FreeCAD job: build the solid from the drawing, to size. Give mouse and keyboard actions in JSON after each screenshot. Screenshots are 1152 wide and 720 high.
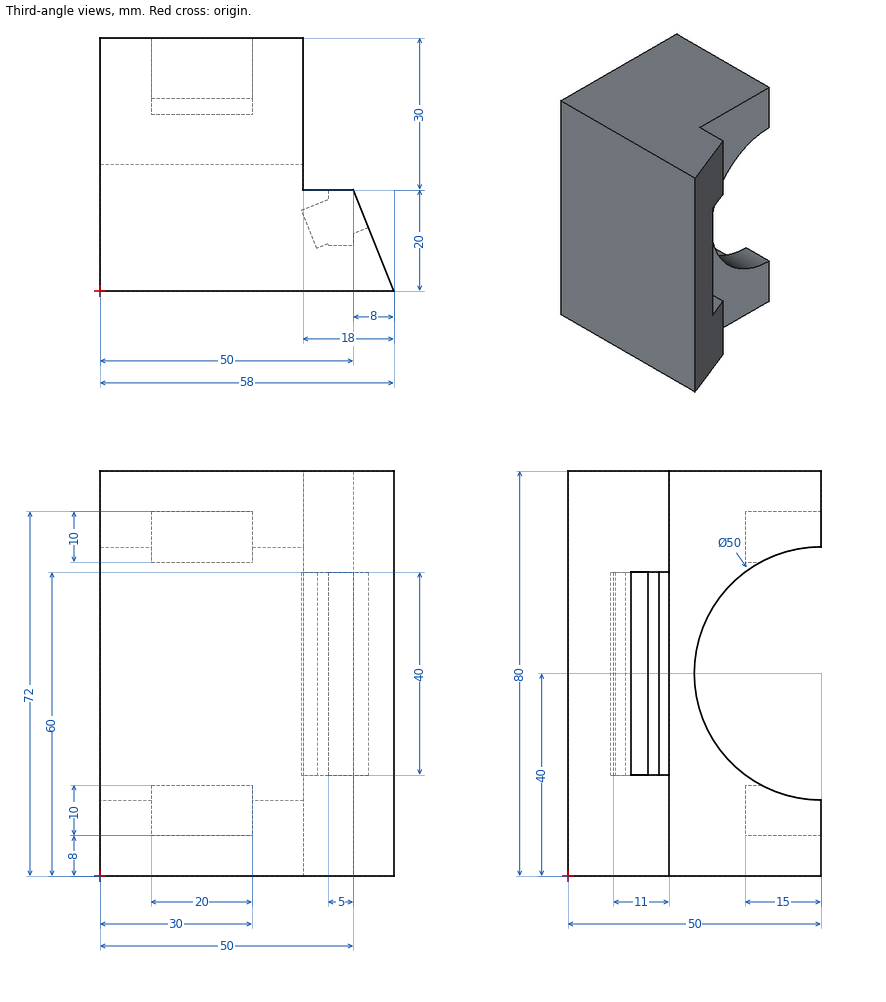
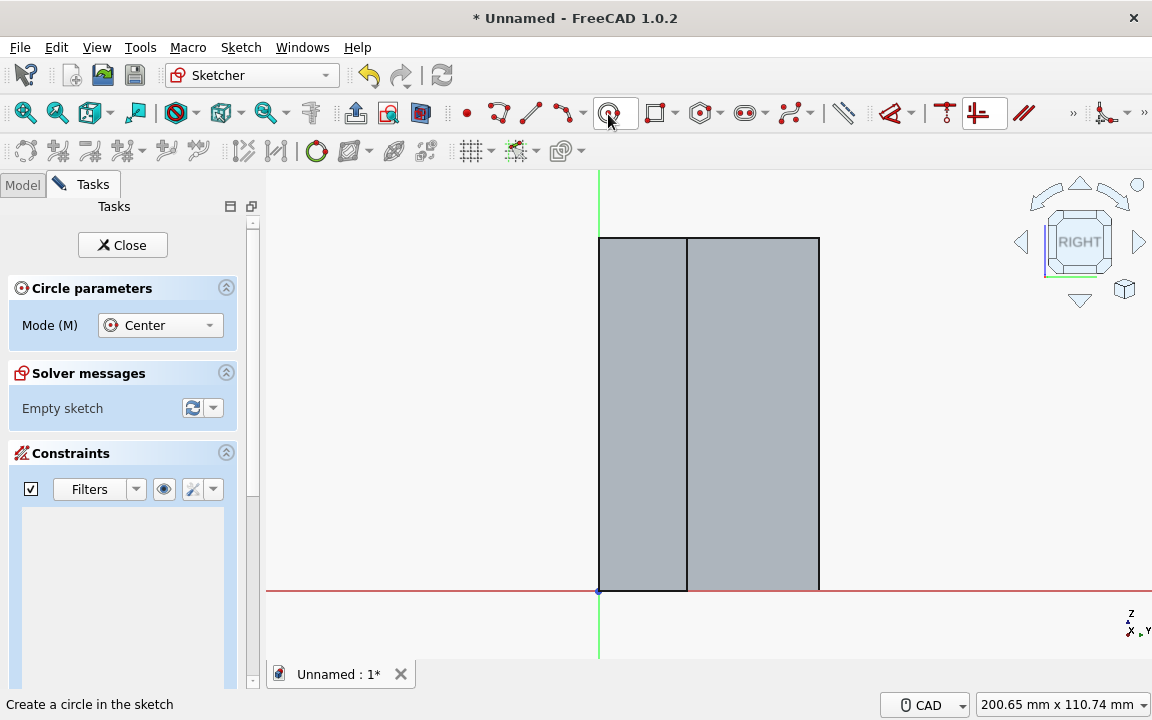
{"action": "left_click", "coordinate": [819, 415]}
{"action": "mouse_move", "coordinate": [897, 336]}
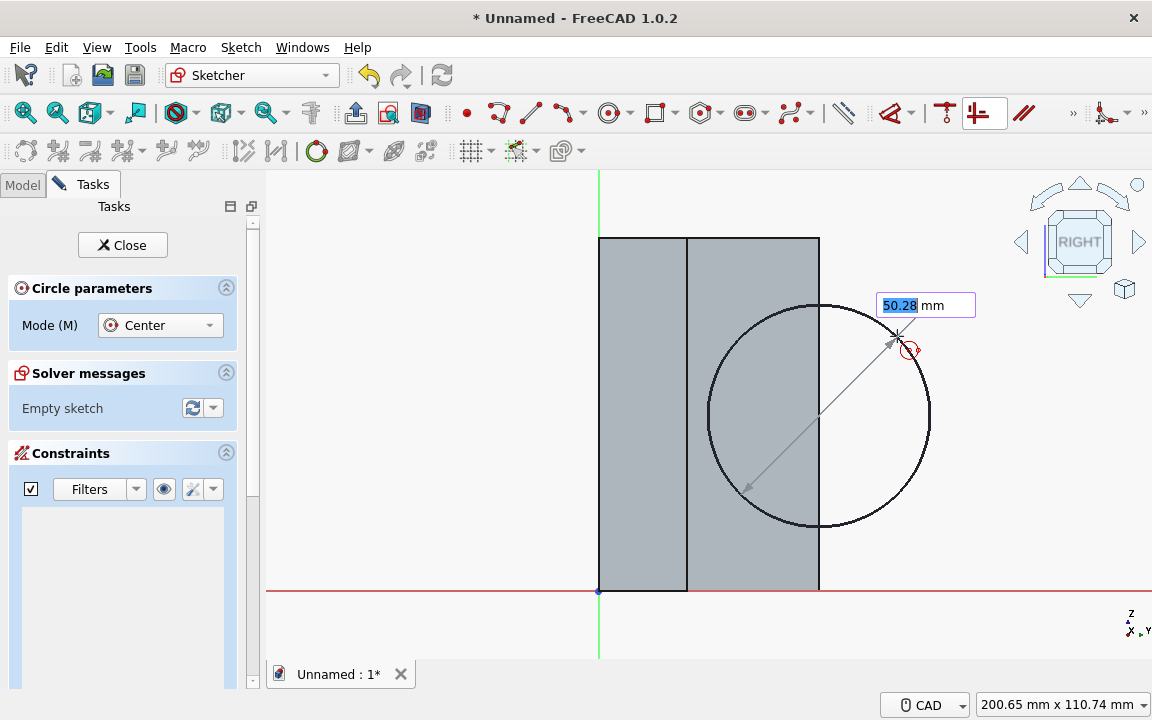
{"action": "type", "text": "50"}
{"action": "key", "text": "Return"}
{"action": "key", "text": "Escape"}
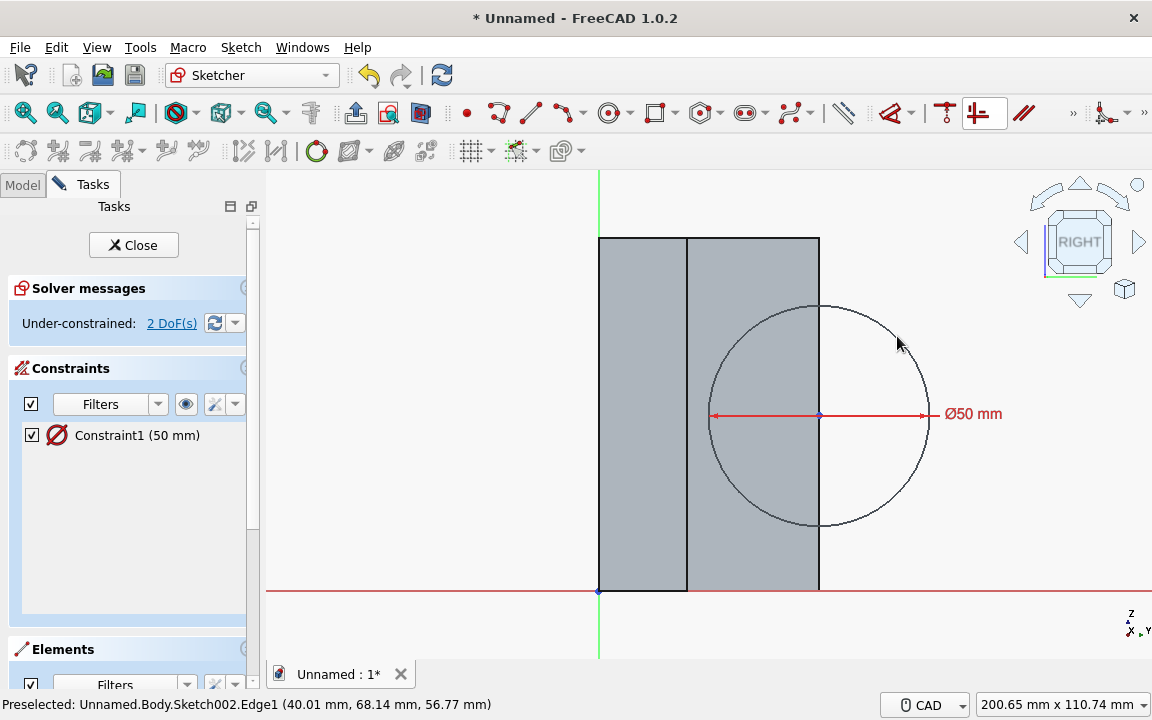
{"action": "left_click", "coordinate": [890, 114]}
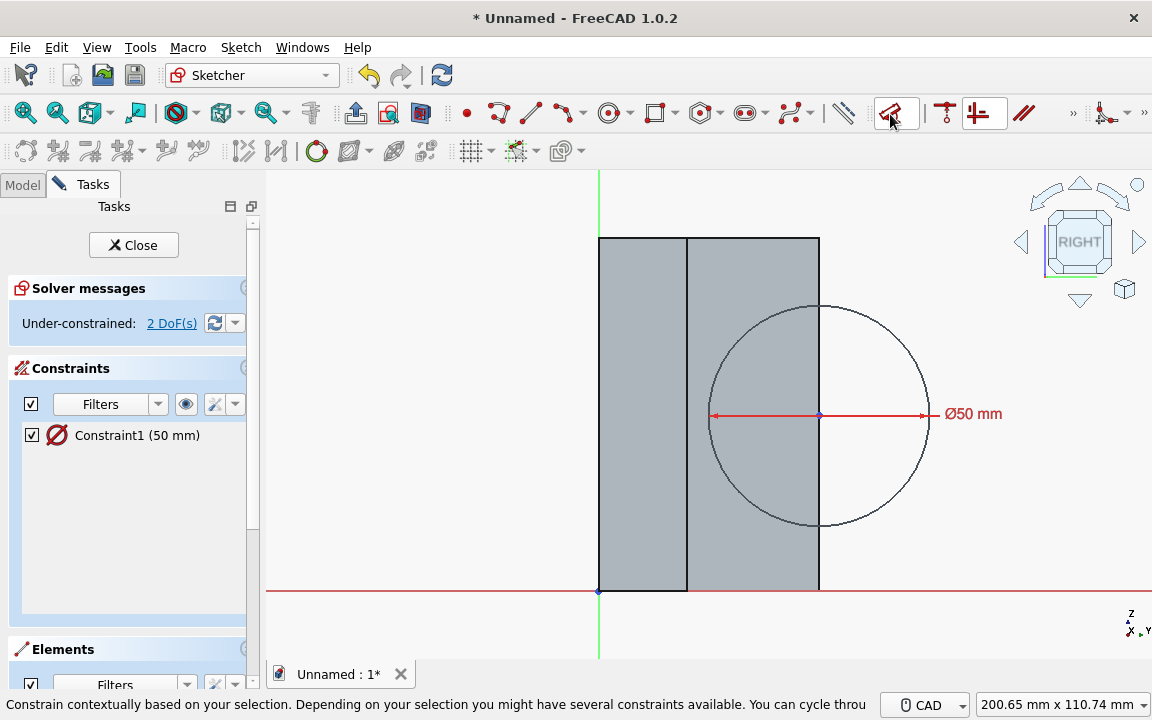
{"action": "left_click", "coordinate": [819, 416]}
{"action": "left_click", "coordinate": [709, 625]}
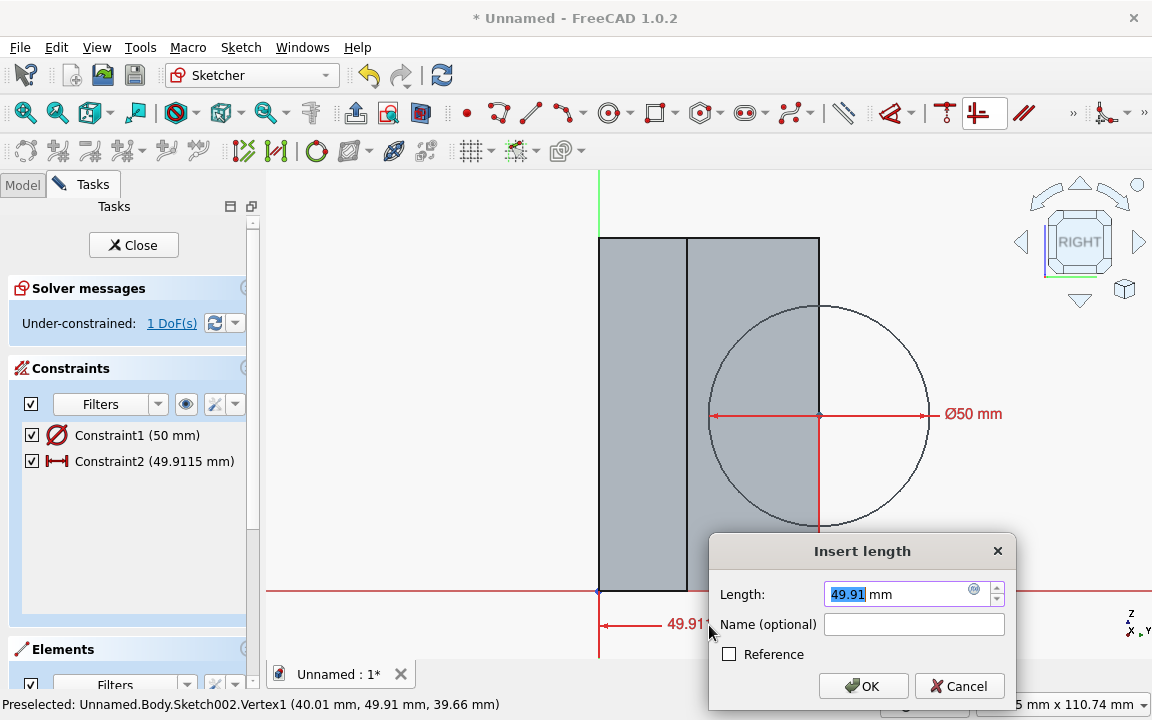
{"action": "type", "text": "50"}
{"action": "key", "text": "Return"}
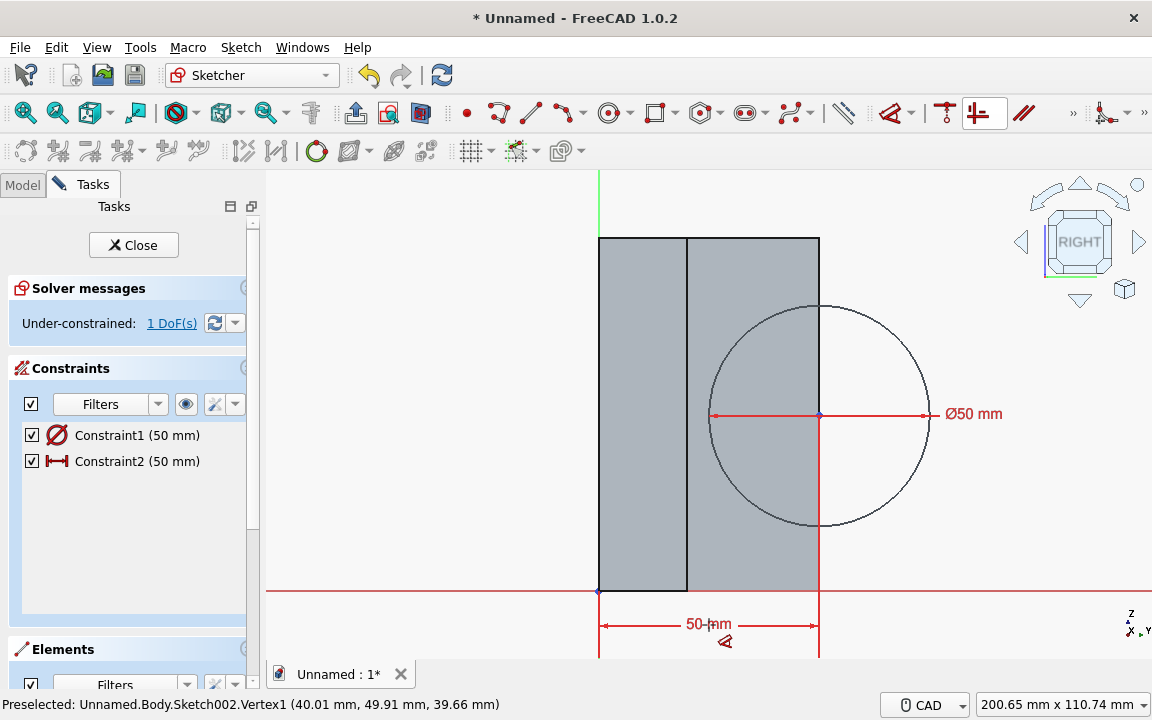
{"action": "left_click", "coordinate": [819, 416]}
{"action": "left_click", "coordinate": [565, 504]}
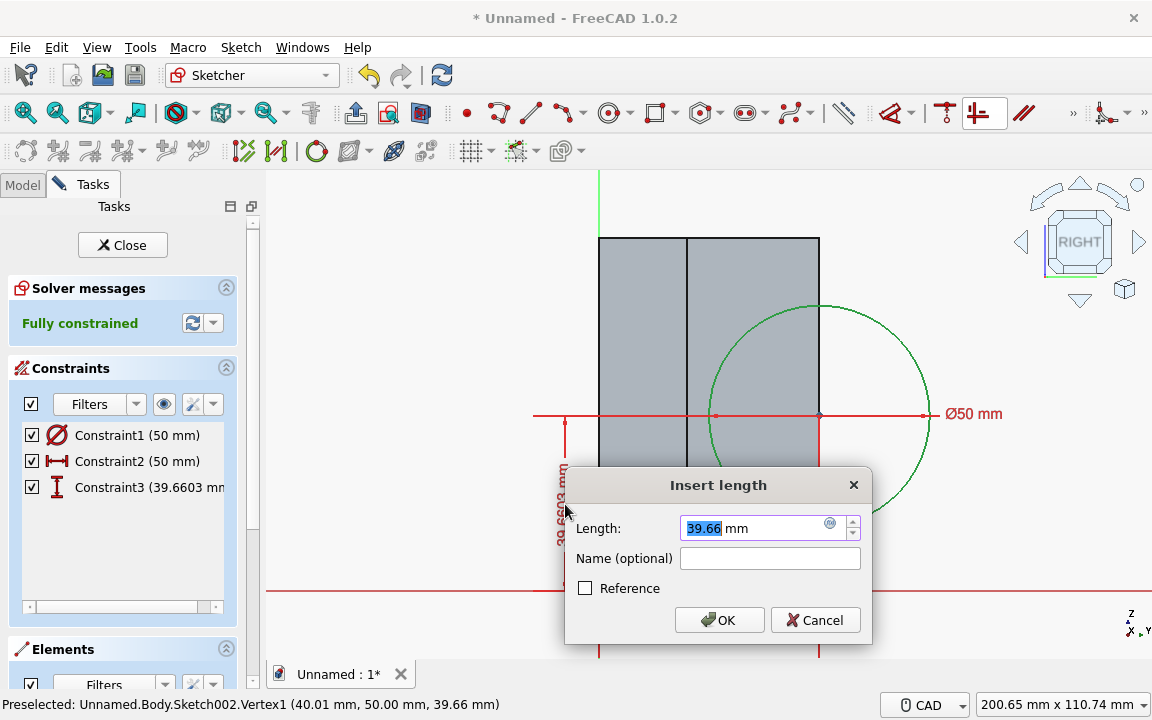
{"action": "type", "text": "40"}
{"action": "key", "text": "Return"}
{"action": "key", "text": "Escape"}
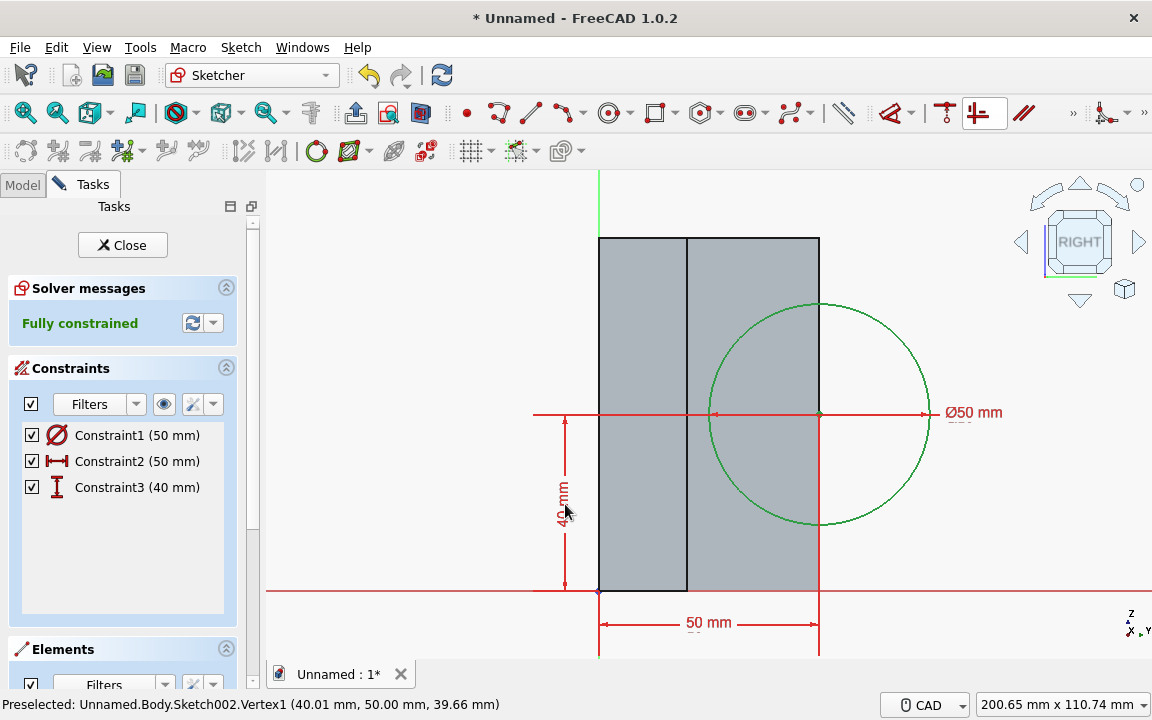
{"action": "left_click", "coordinate": [123, 245]}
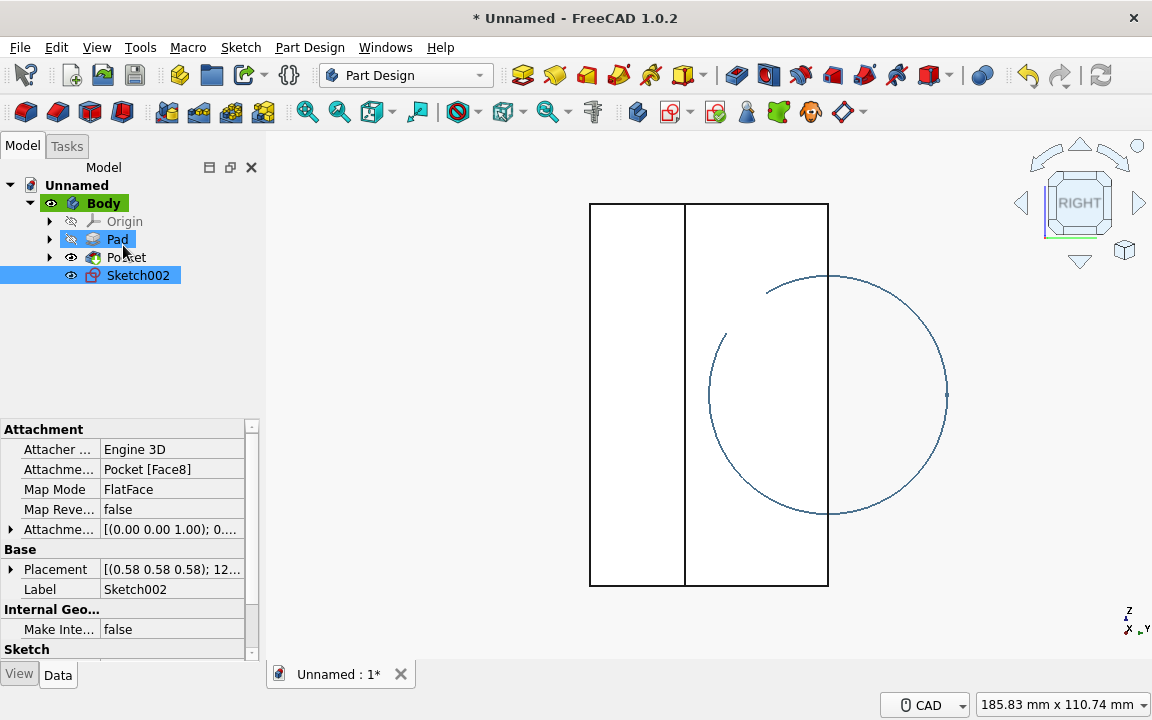
{"action": "left_click", "coordinate": [738, 76]}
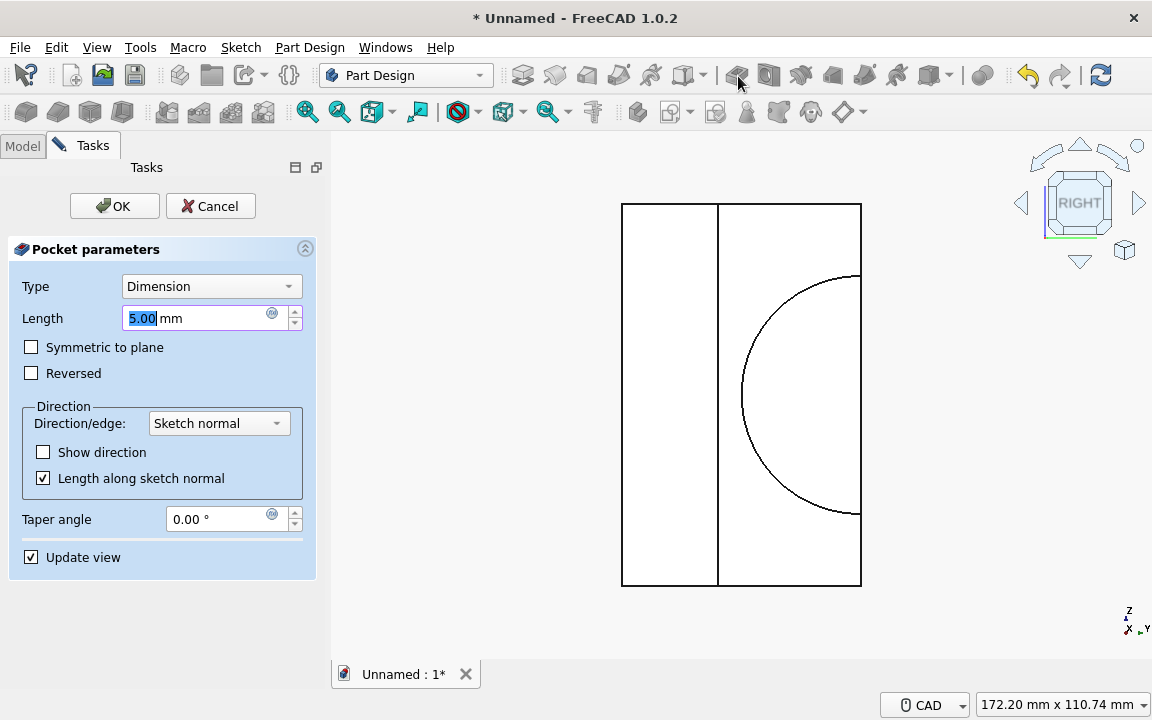
{"action": "left_click", "coordinate": [212, 286]}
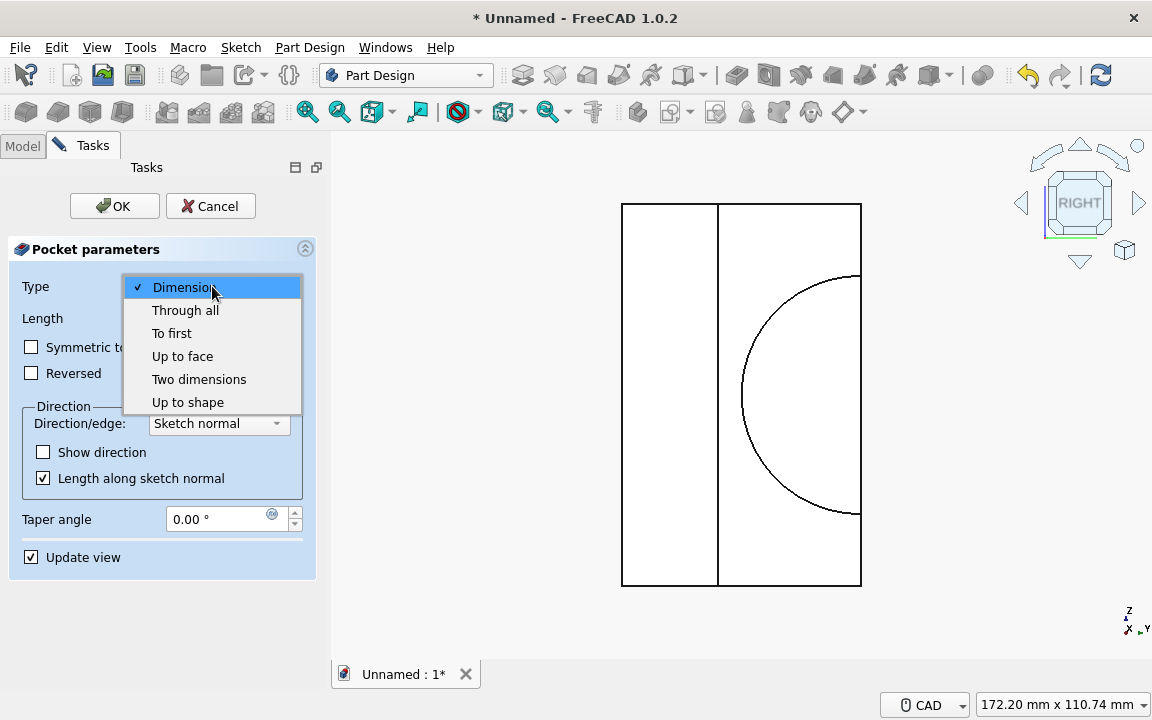
{"action": "left_click", "coordinate": [212, 310]}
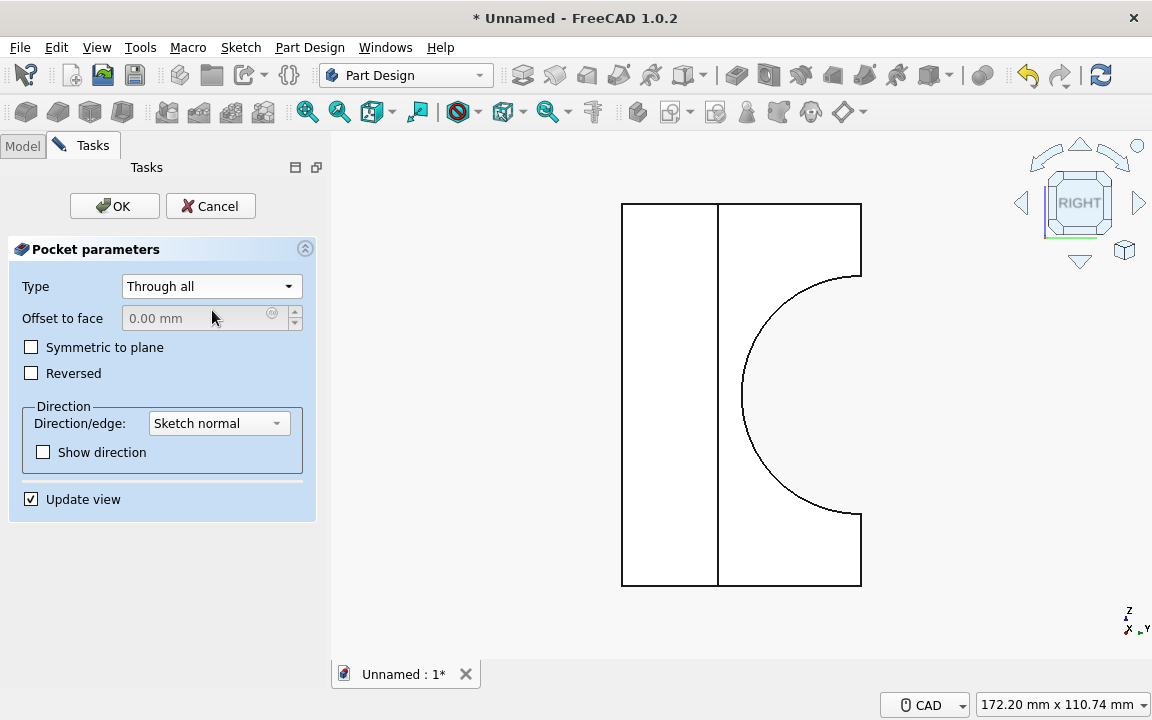
{"action": "left_click", "coordinate": [115, 206]}